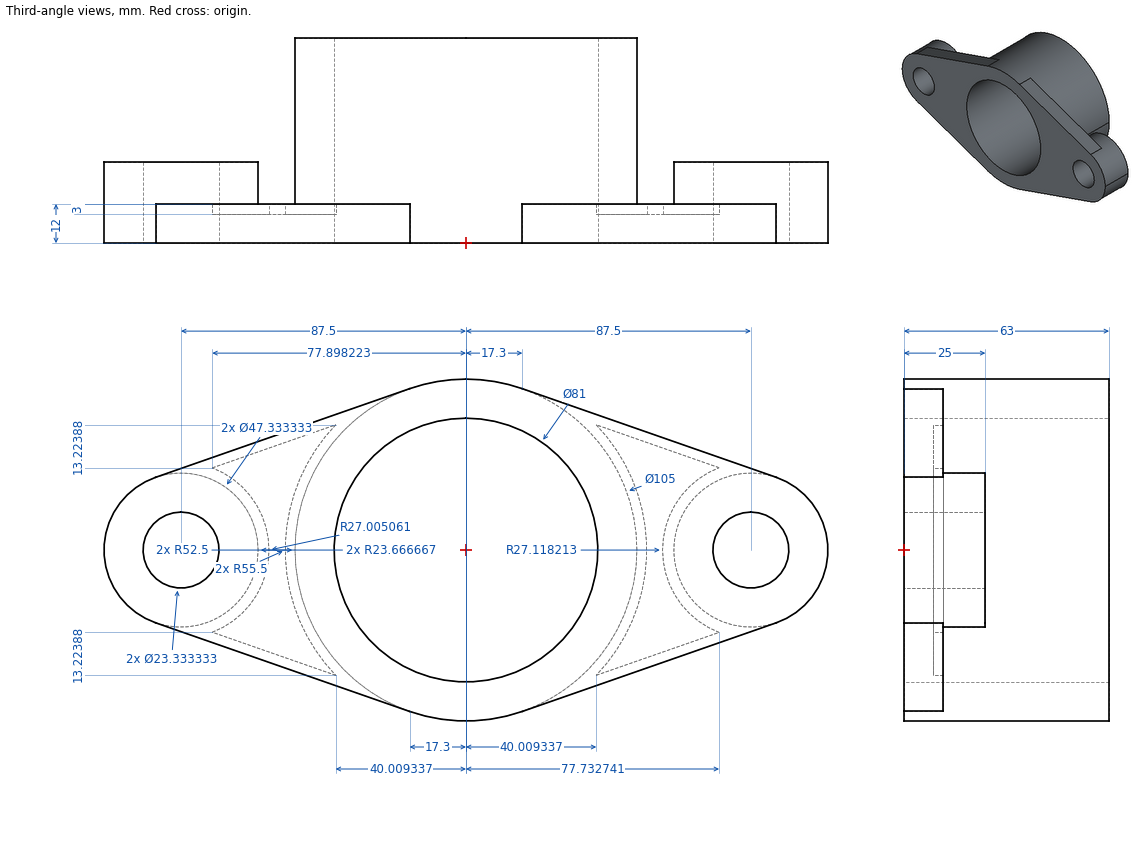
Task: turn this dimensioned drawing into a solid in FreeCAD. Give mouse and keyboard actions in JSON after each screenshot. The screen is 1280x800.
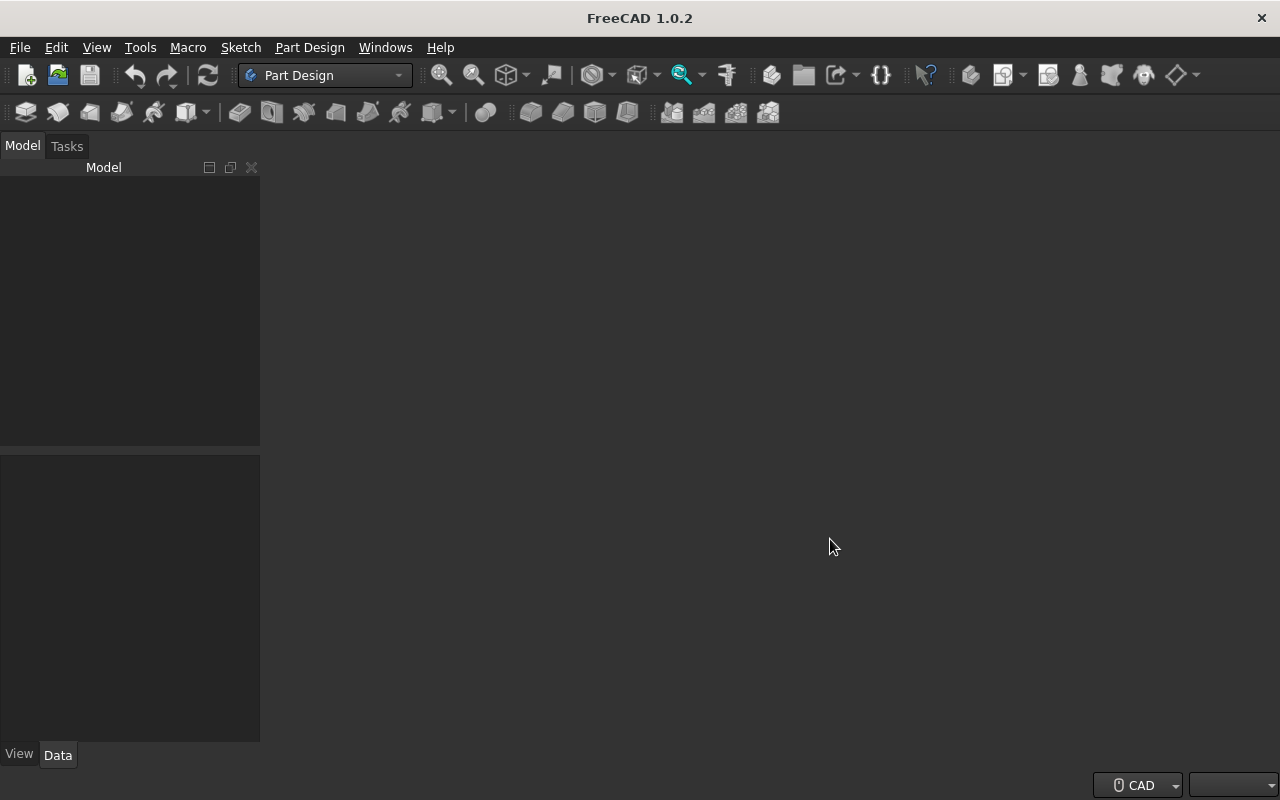
{"action": "key", "text": "ctrl+n"}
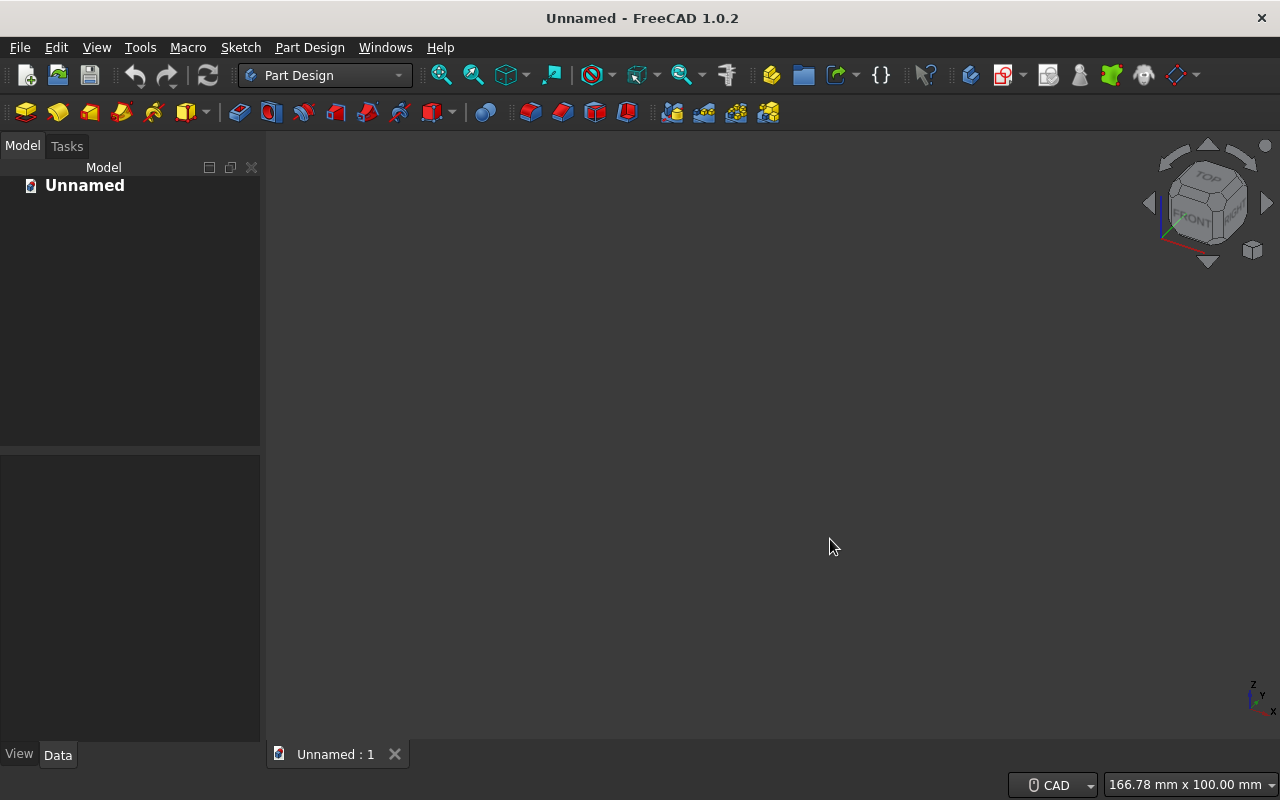
{"action": "left_click", "coordinate": [1004, 76]}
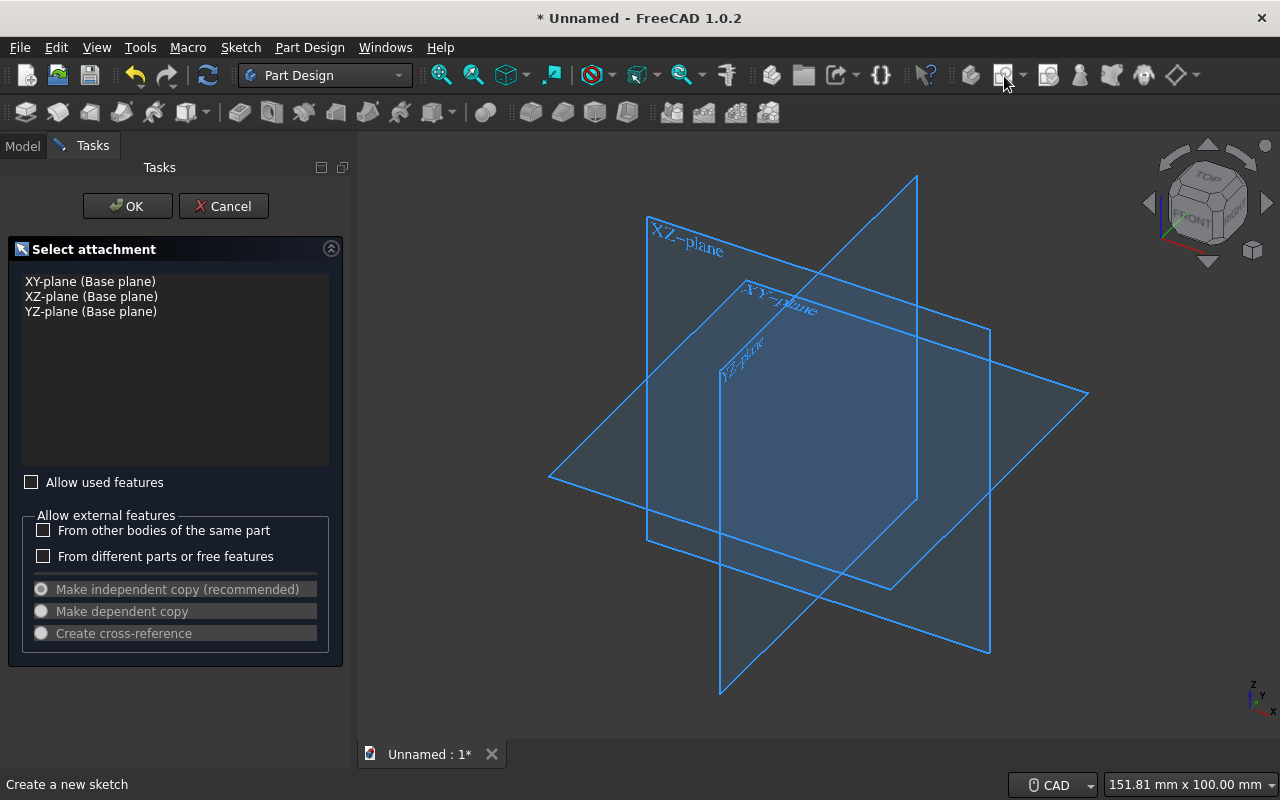
{"action": "left_click", "coordinate": [82, 296]}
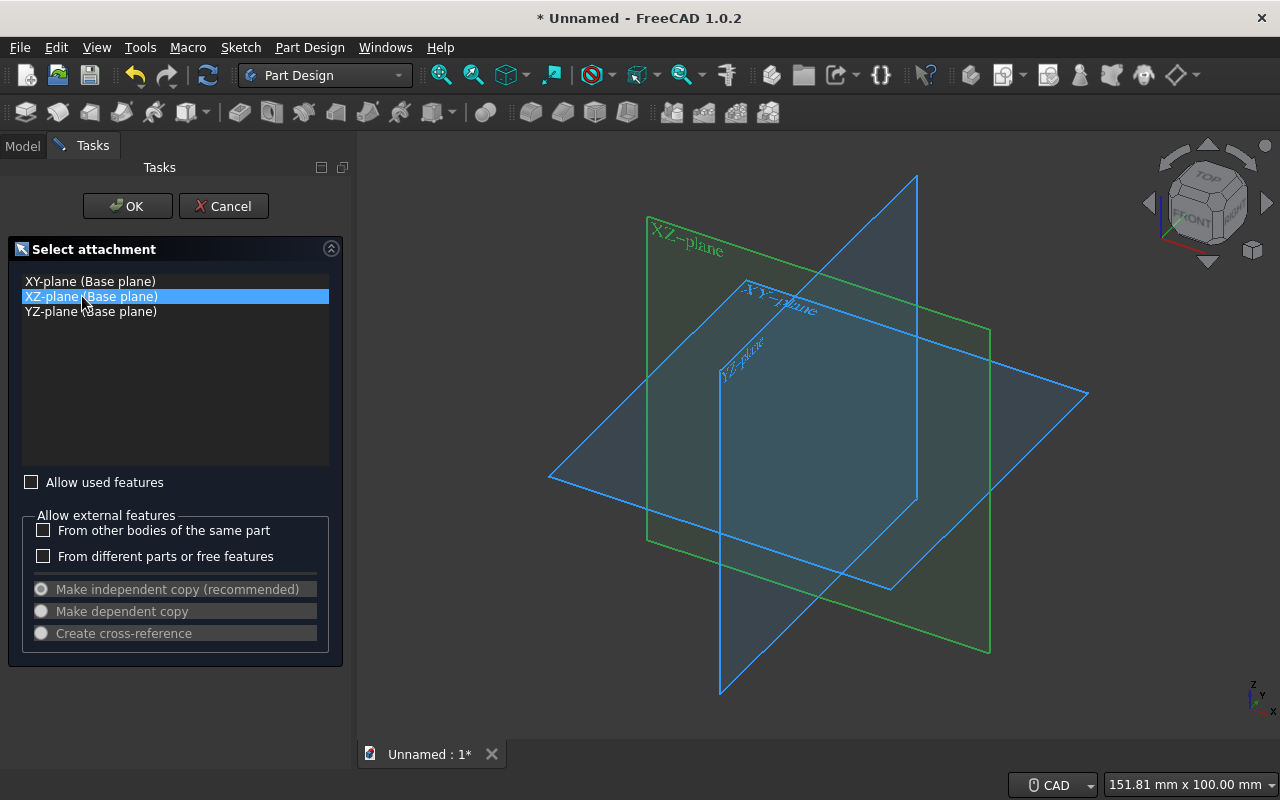
{"action": "left_click", "coordinate": [128, 206]}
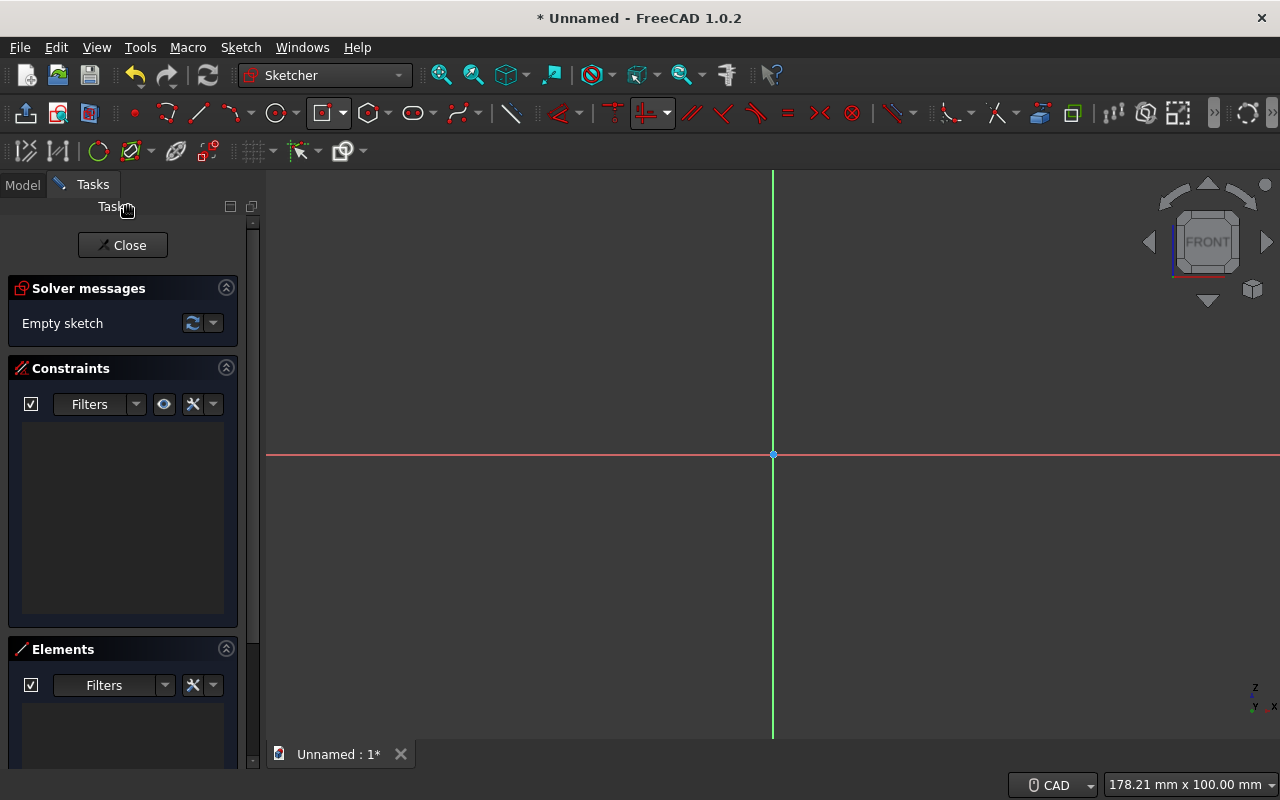
{"action": "scroll", "coordinate": [621, 454], "scroll_direction": "down", "scroll_amount": 3}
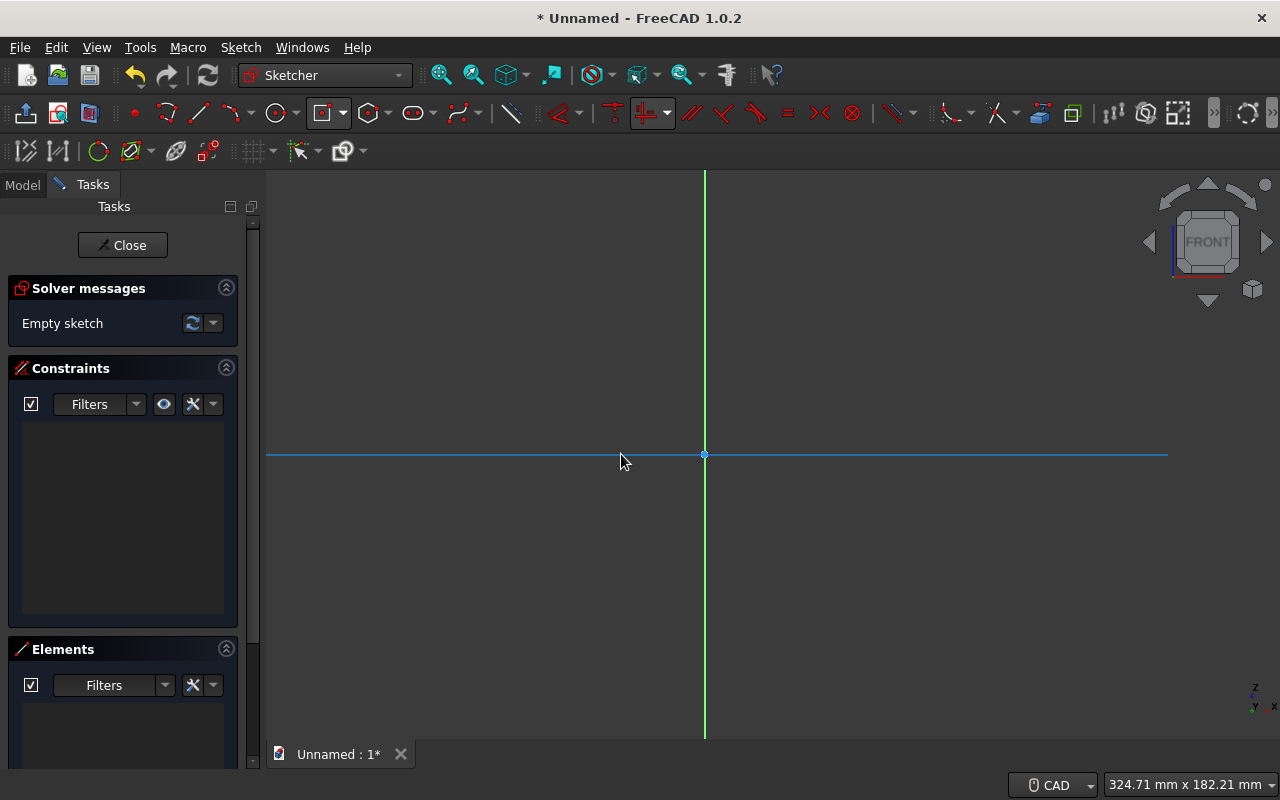
{"action": "left_click", "coordinate": [276, 114]}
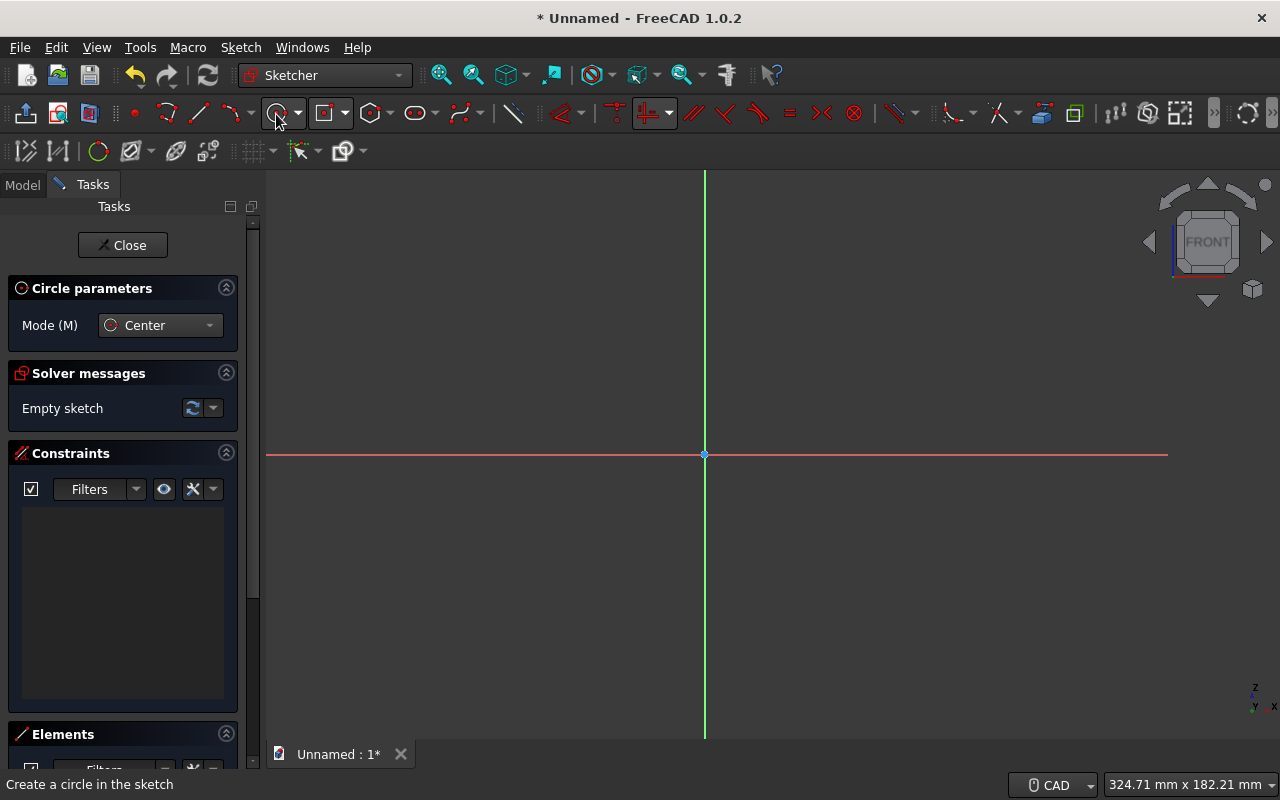
{"action": "left_click", "coordinate": [705, 454]}
{"action": "left_click", "coordinate": [821, 339]}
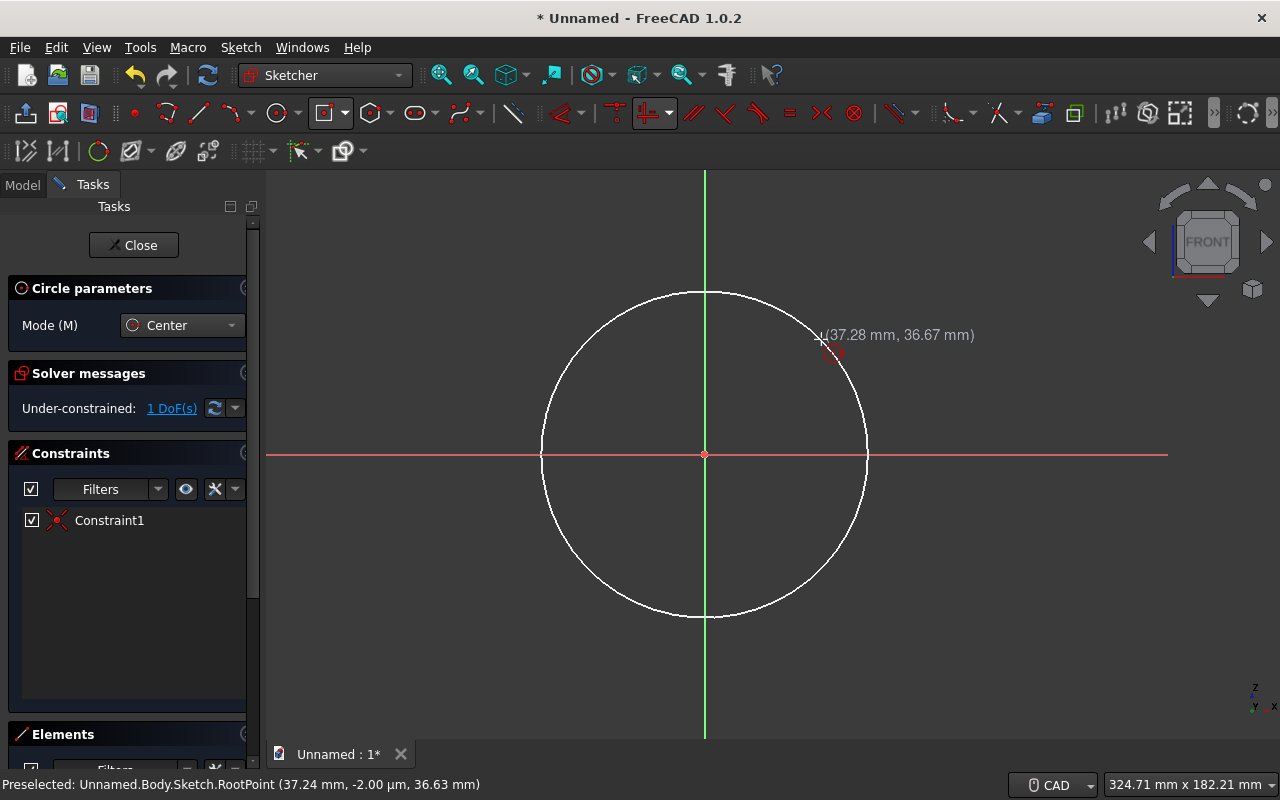
{"action": "left_click", "coordinate": [705, 454]}
{"action": "left_click", "coordinate": [794, 365]}
{"action": "key", "text": "Escape"}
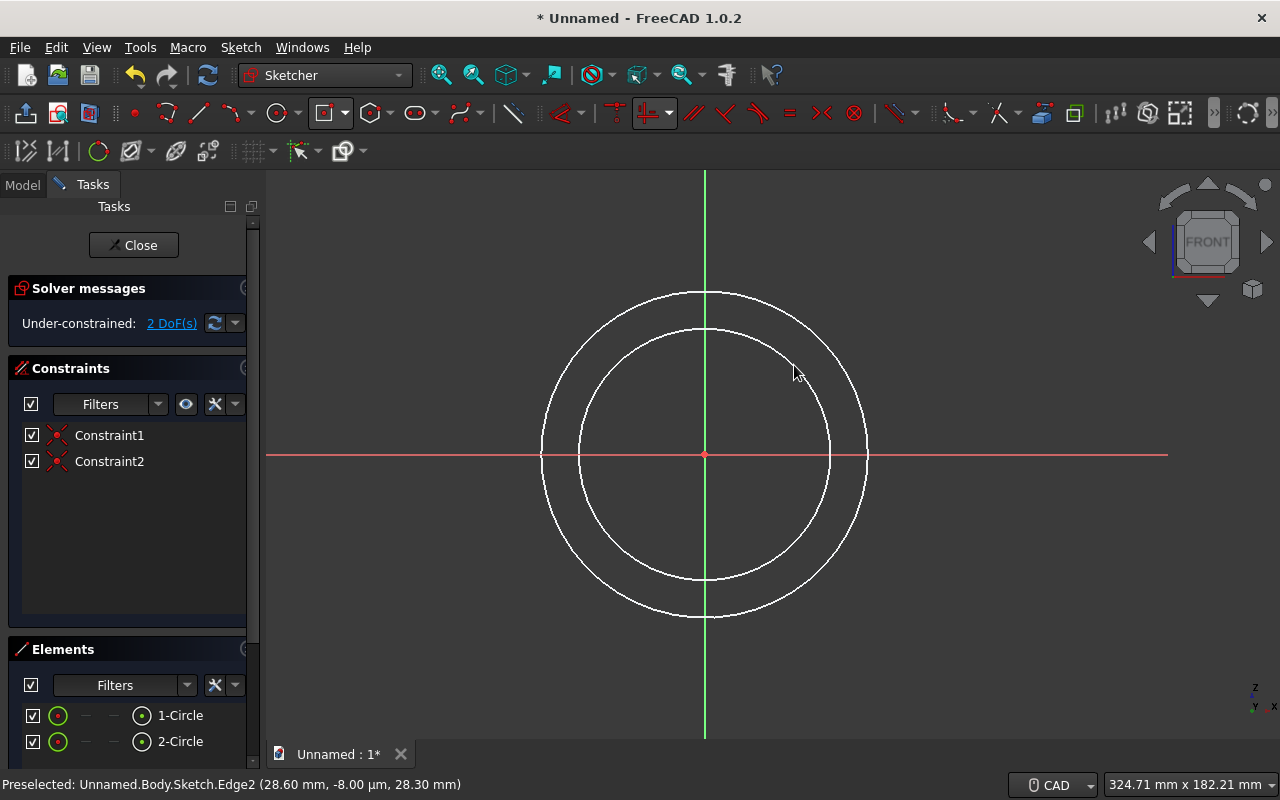
{"action": "left_click", "coordinate": [820, 339]}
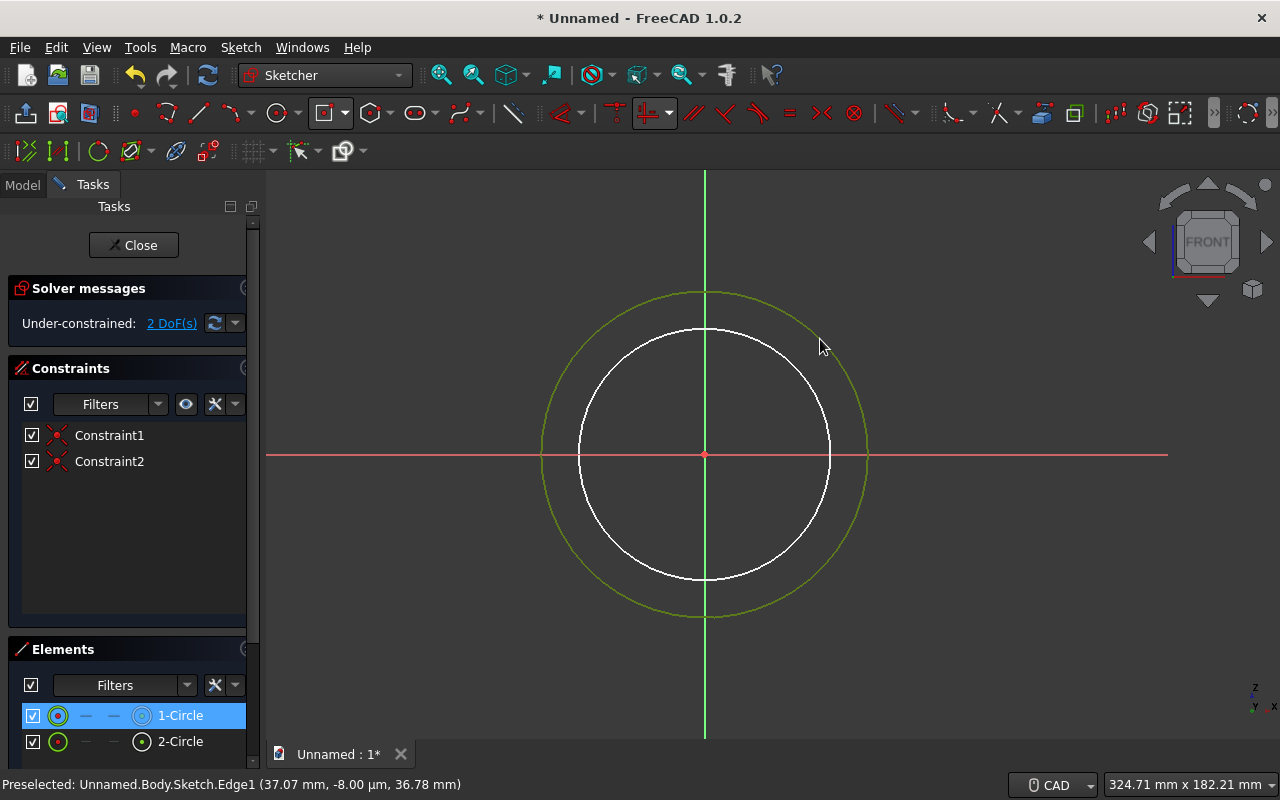
{"action": "left_click", "coordinate": [584, 114]}